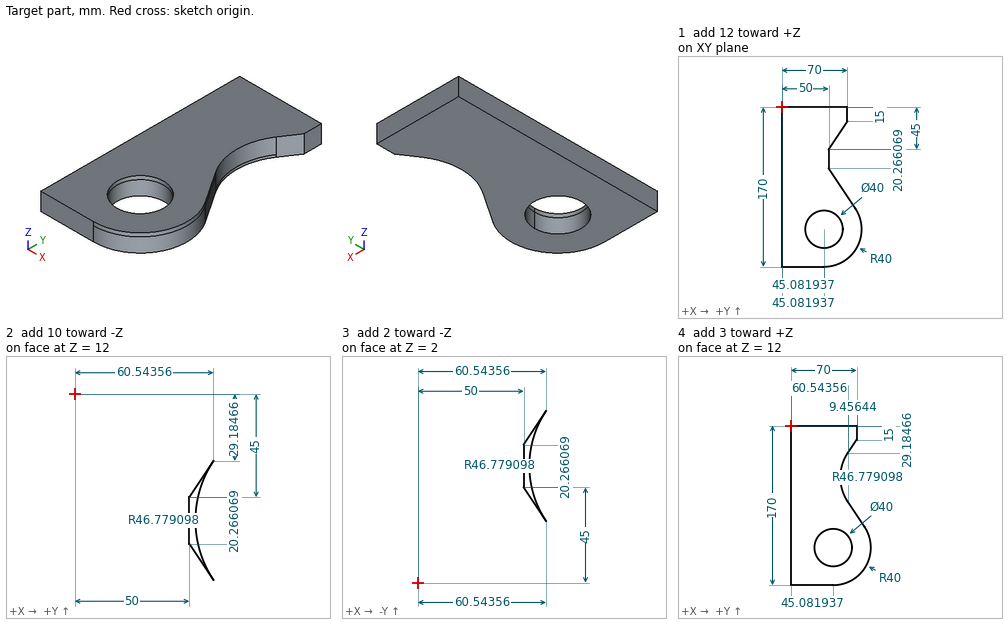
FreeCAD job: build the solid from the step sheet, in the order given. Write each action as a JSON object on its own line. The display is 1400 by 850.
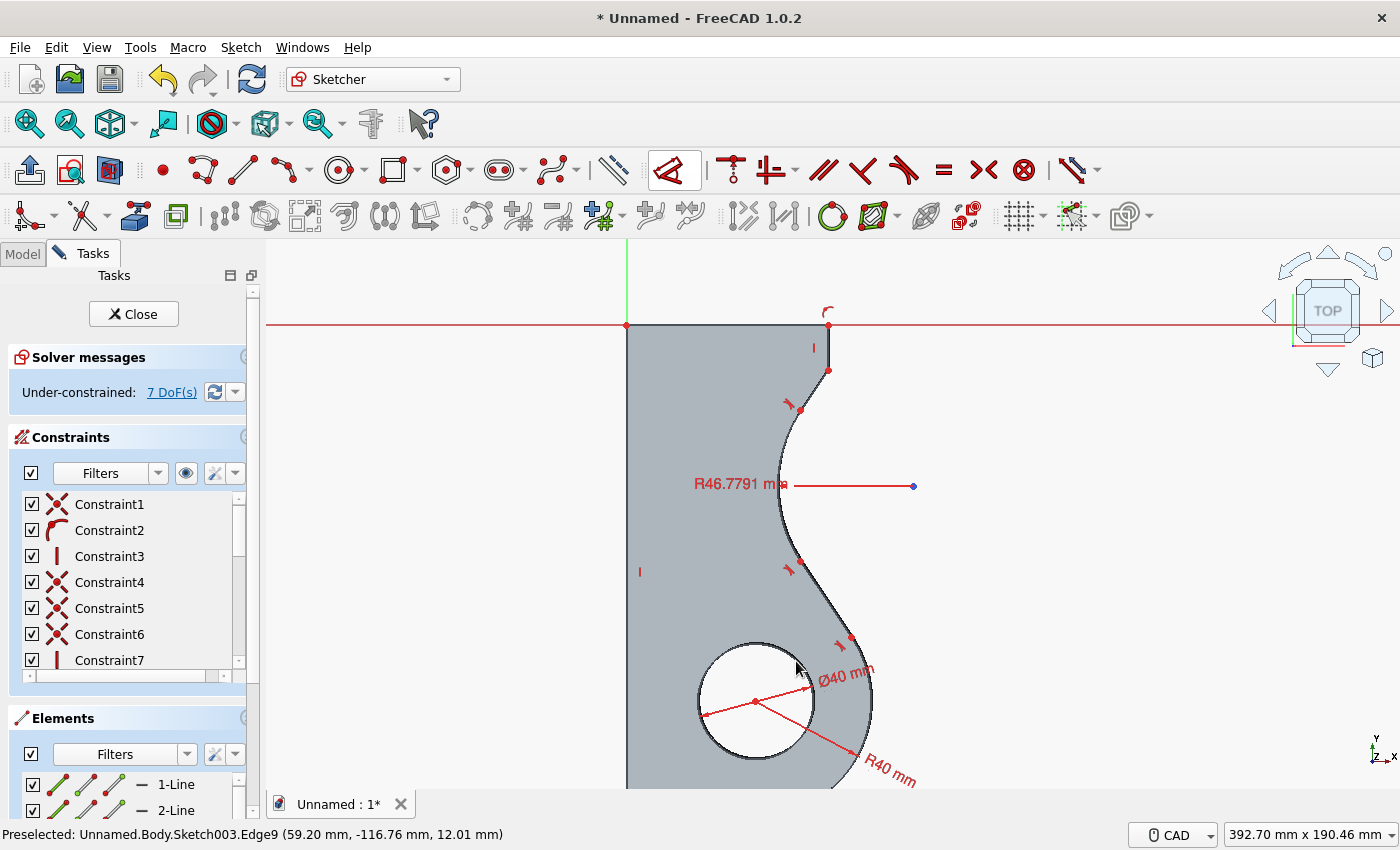
{"action": "left_click", "coordinate": [828, 357]}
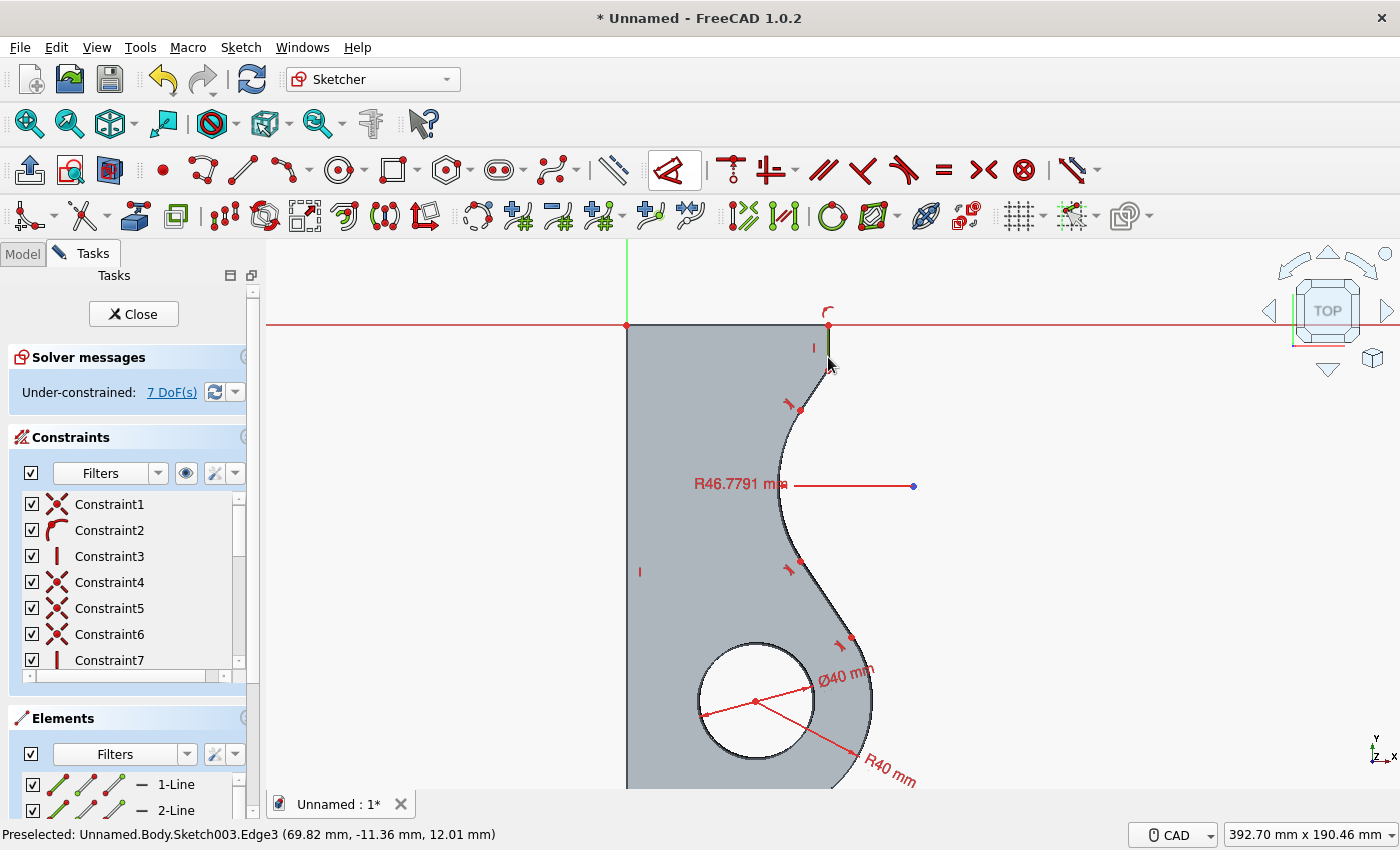
{"action": "left_click", "coordinate": [696, 170]}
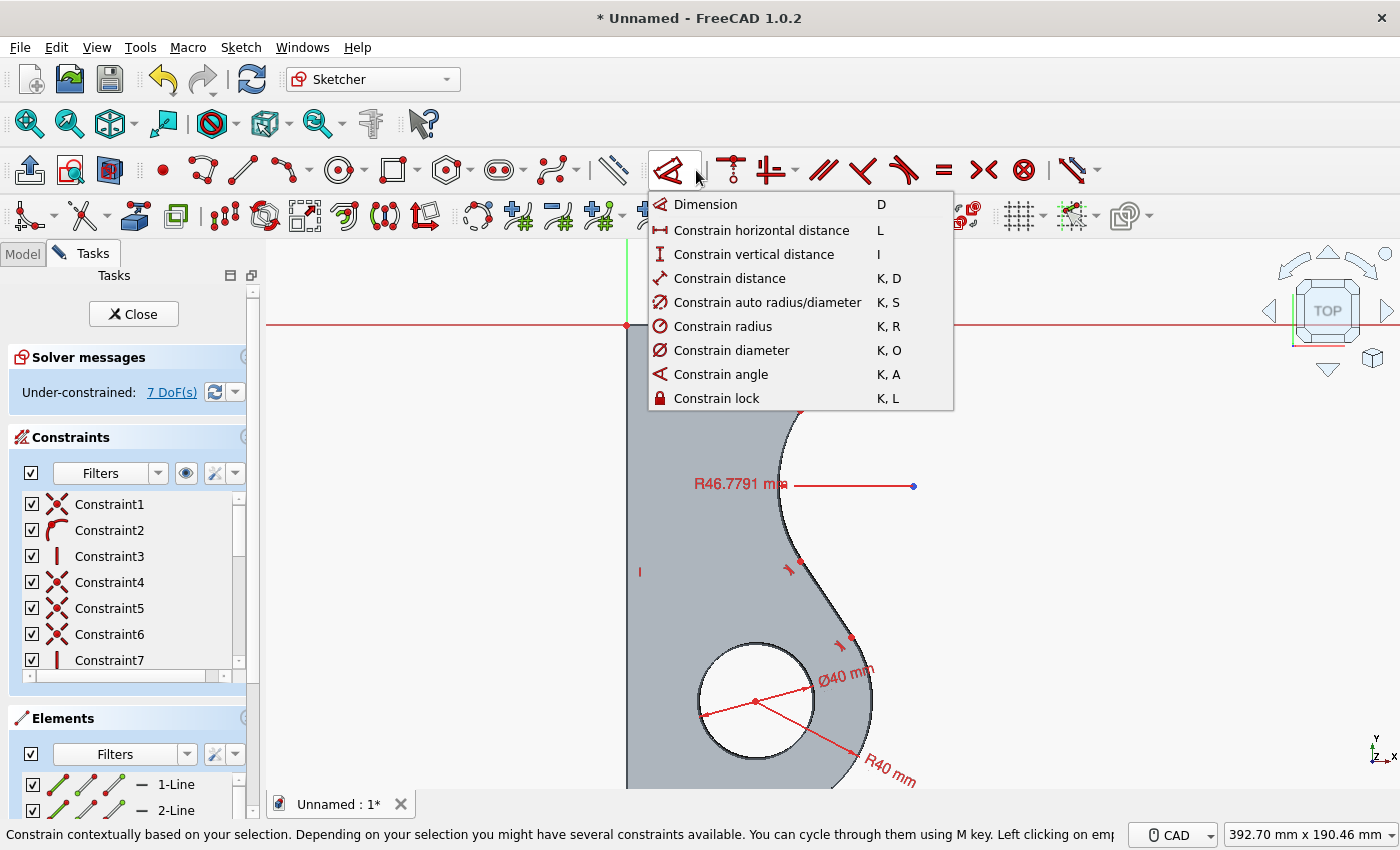
{"action": "left_click", "coordinate": [801, 254]}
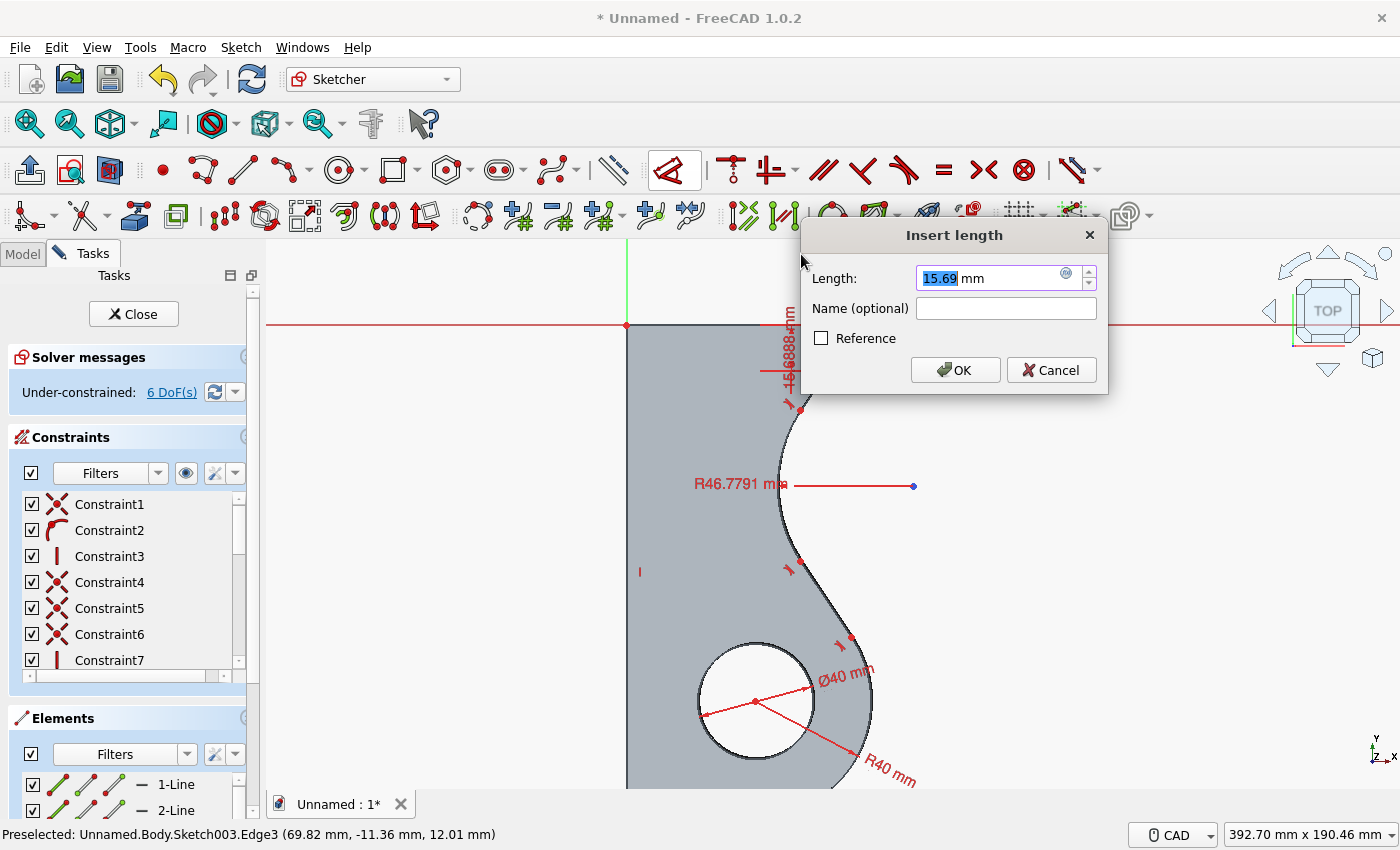
{"action": "type", "text": "15"}
{"action": "key", "text": "Return"}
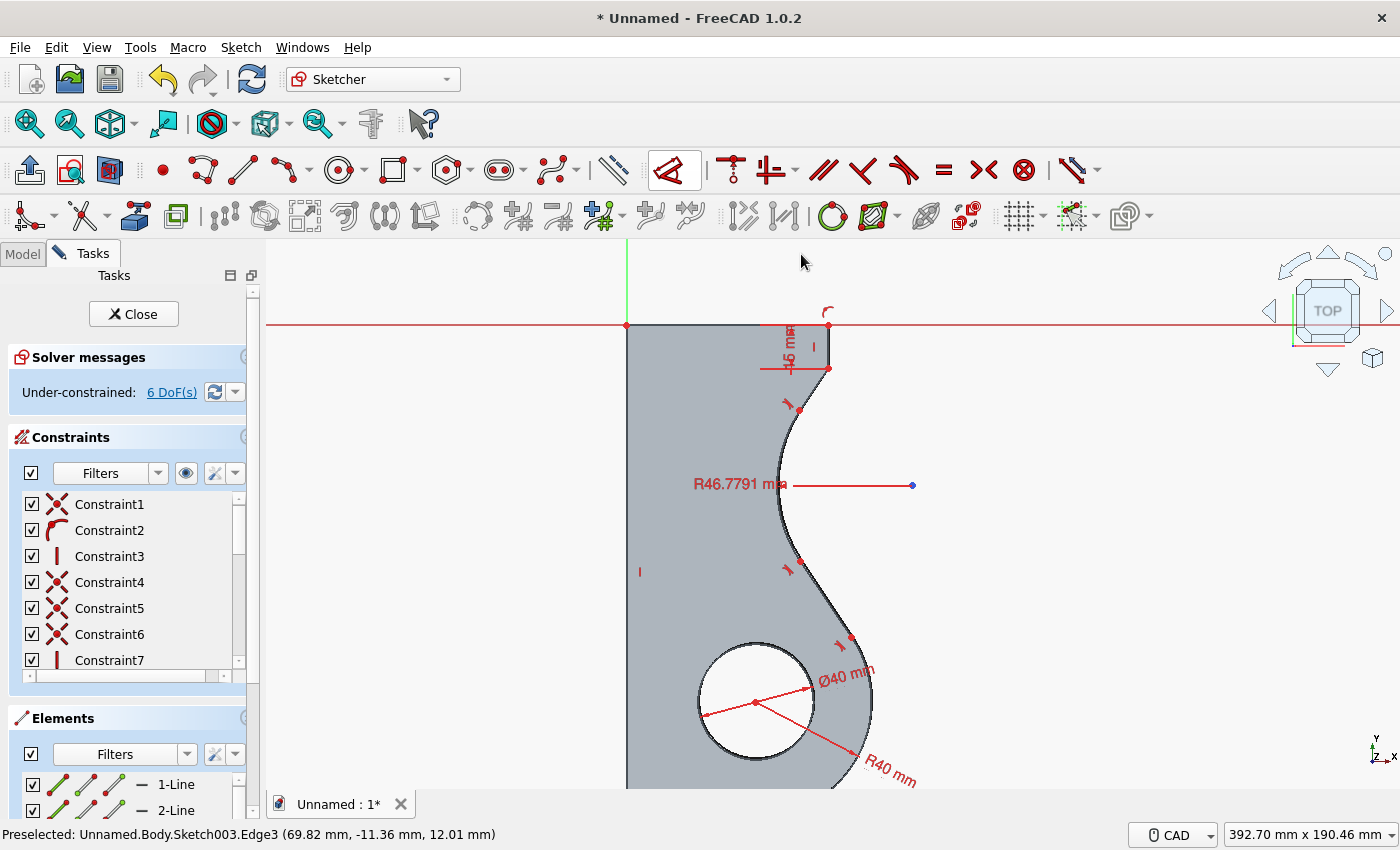
{"action": "left_click", "coordinate": [768, 325]}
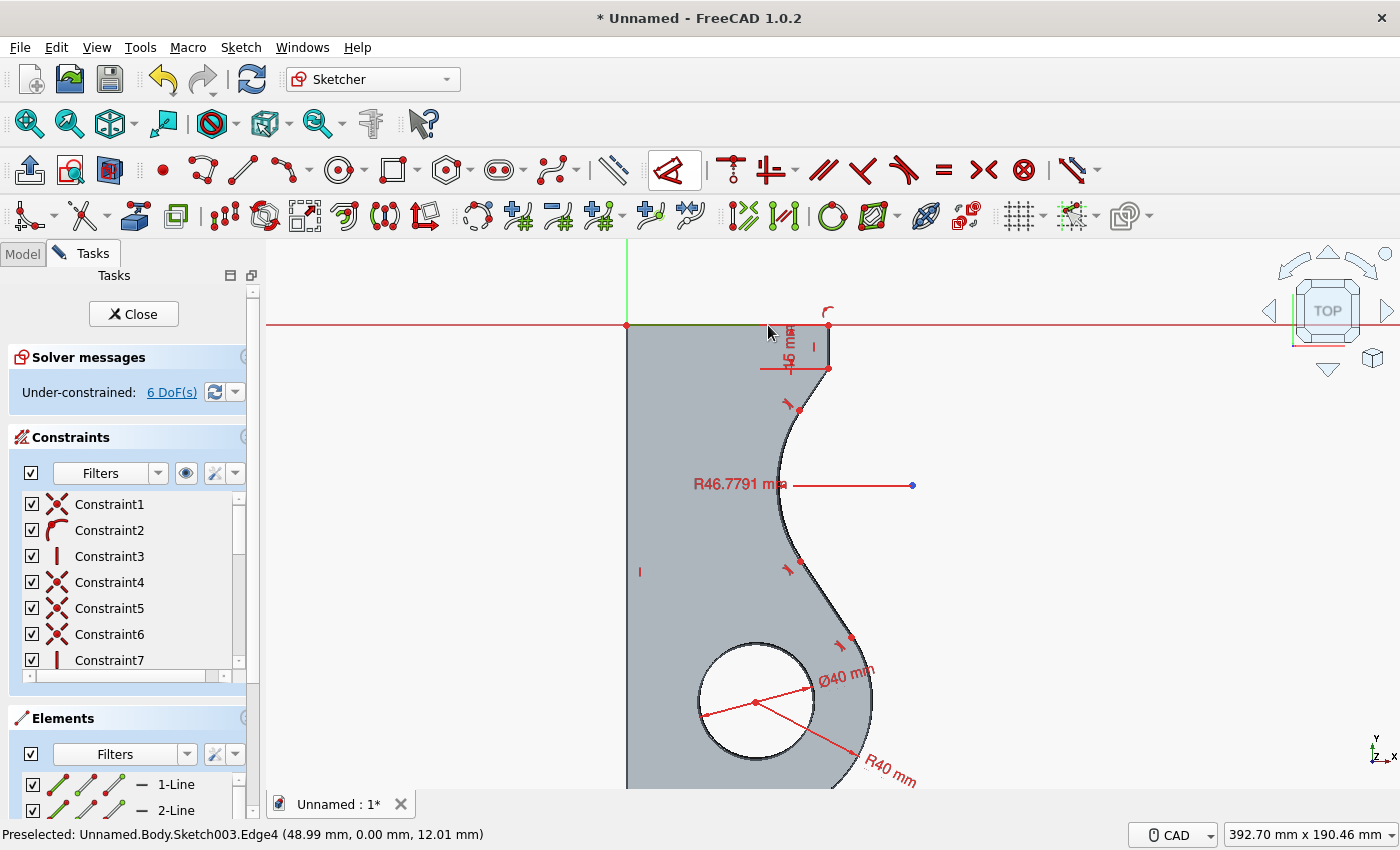
{"action": "left_click", "coordinate": [696, 170]}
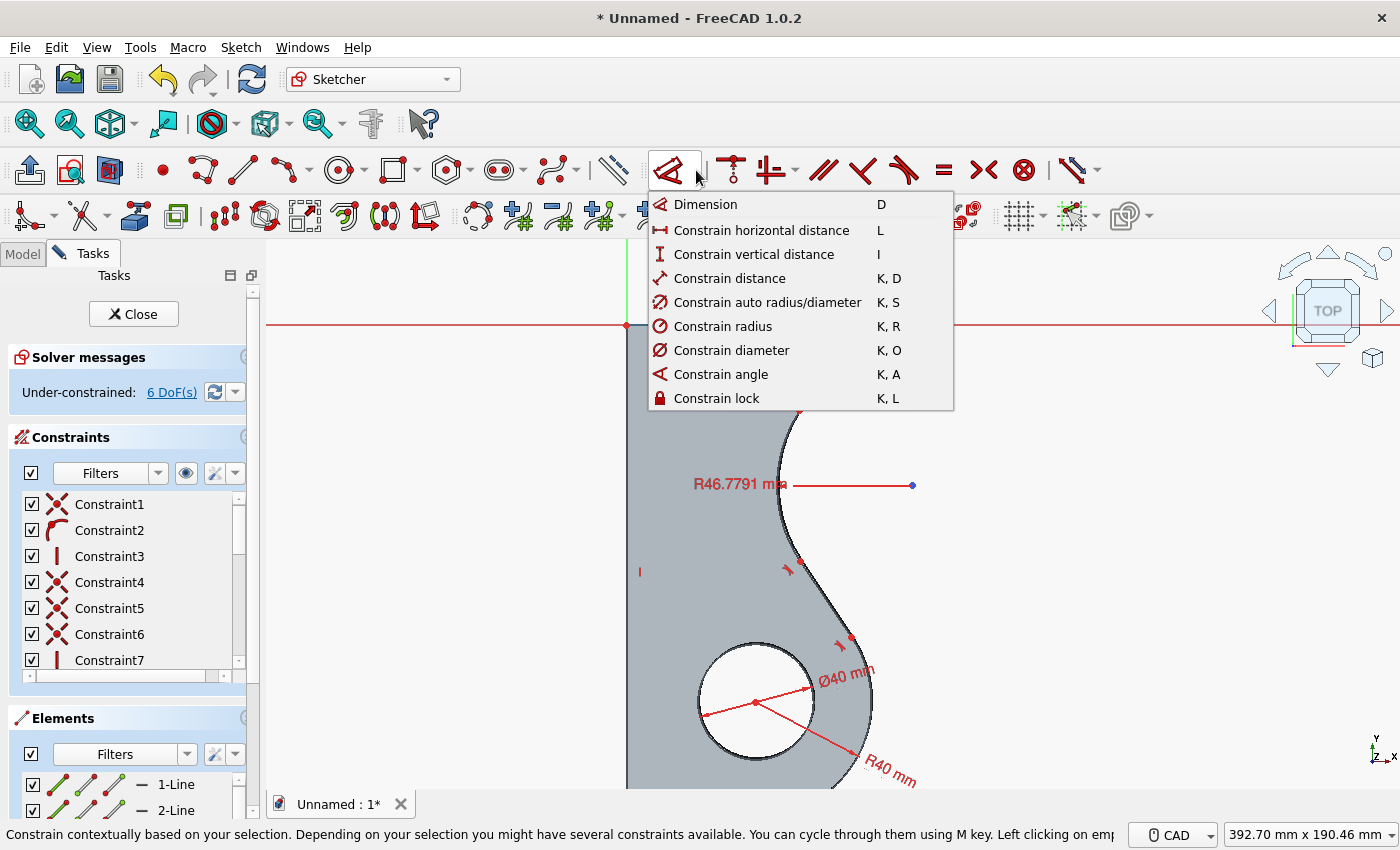
{"action": "left_click", "coordinate": [801, 230]}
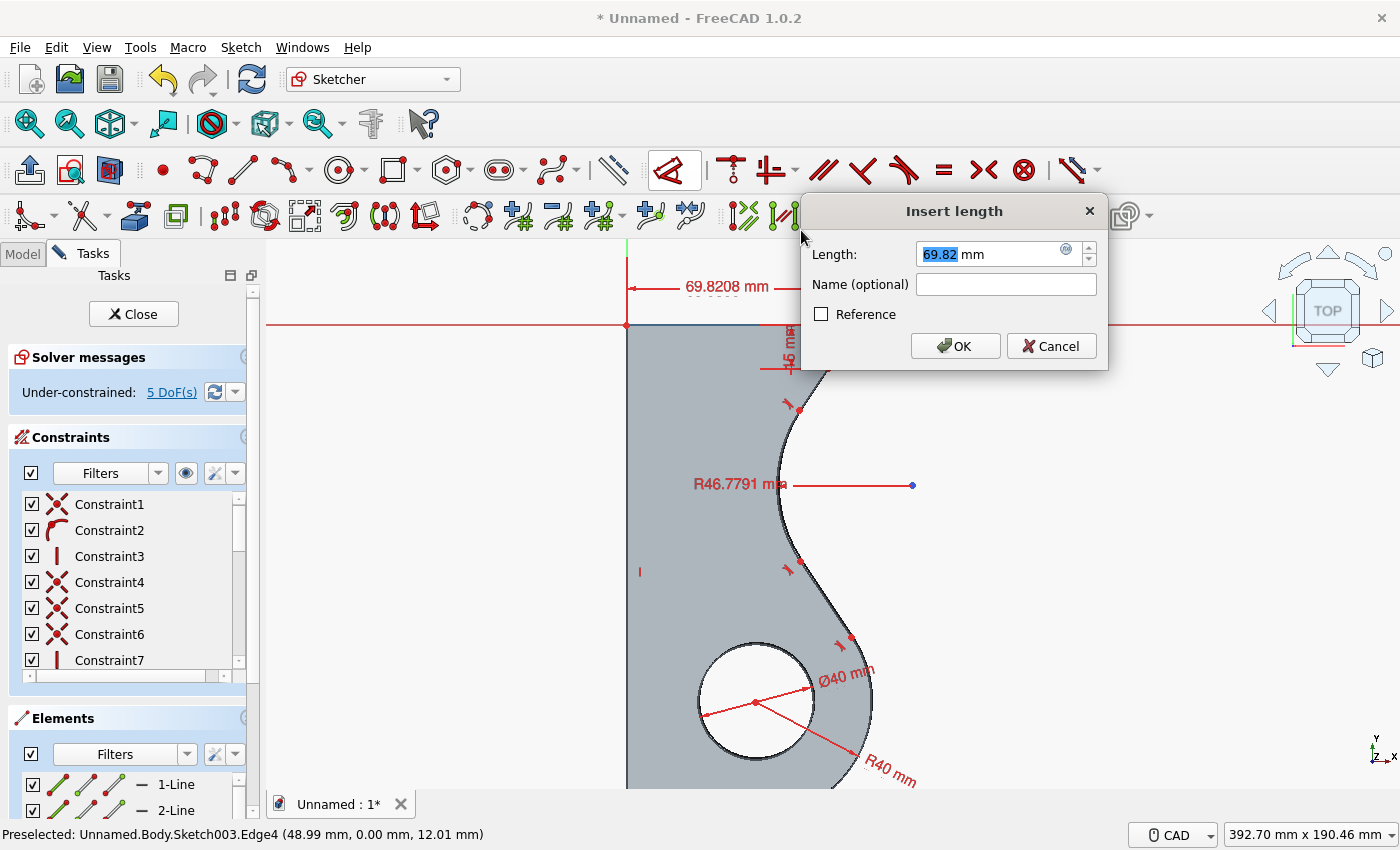
{"action": "type", "text": "70"}
{"action": "key", "text": "Return"}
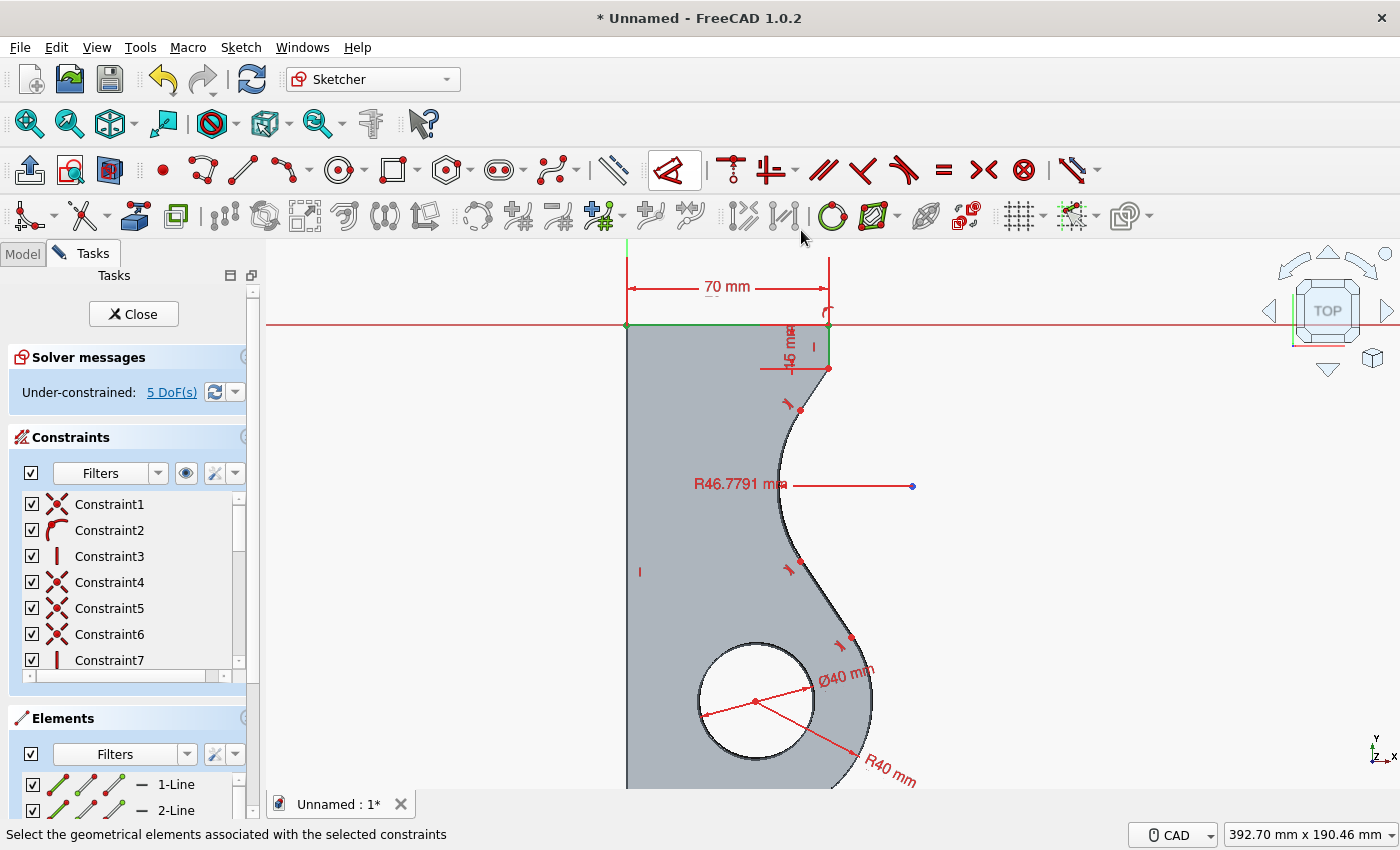
{"action": "left_click", "coordinate": [627, 473]}